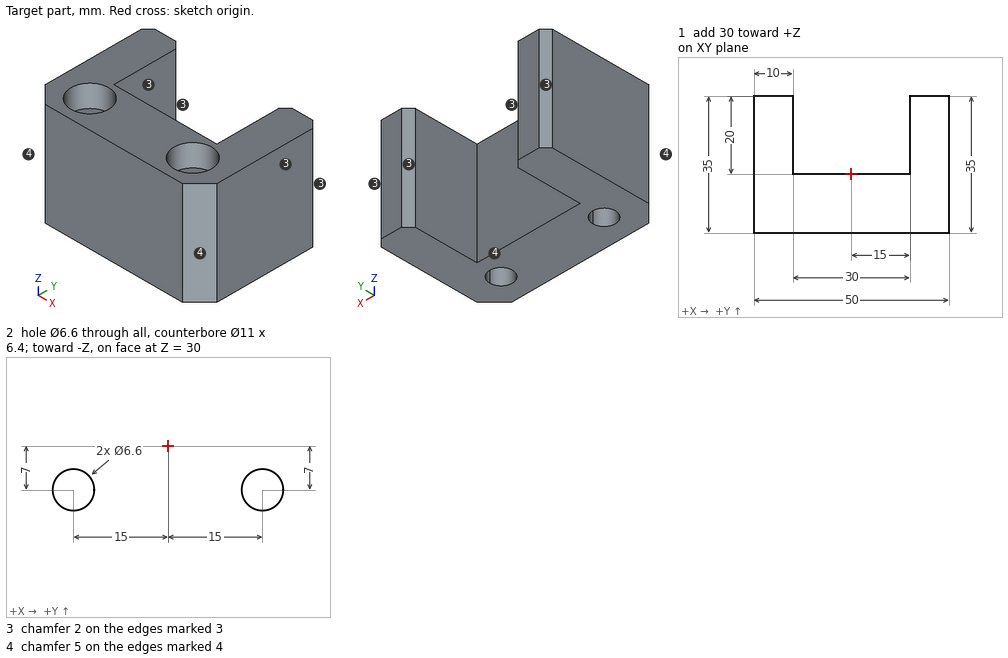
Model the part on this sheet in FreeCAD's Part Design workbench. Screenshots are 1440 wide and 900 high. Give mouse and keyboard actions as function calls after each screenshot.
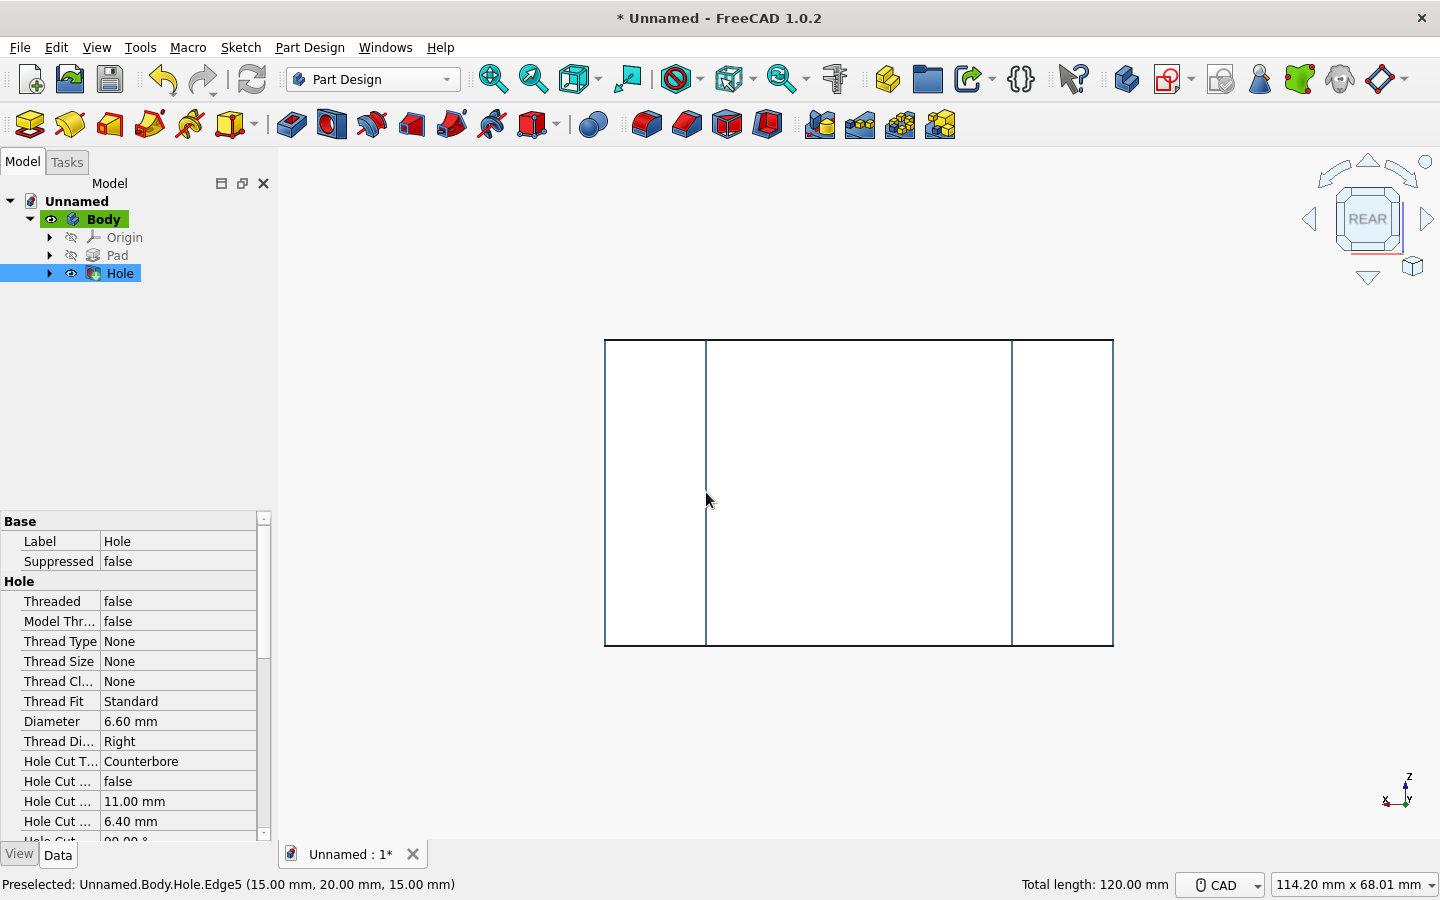
click(688, 124)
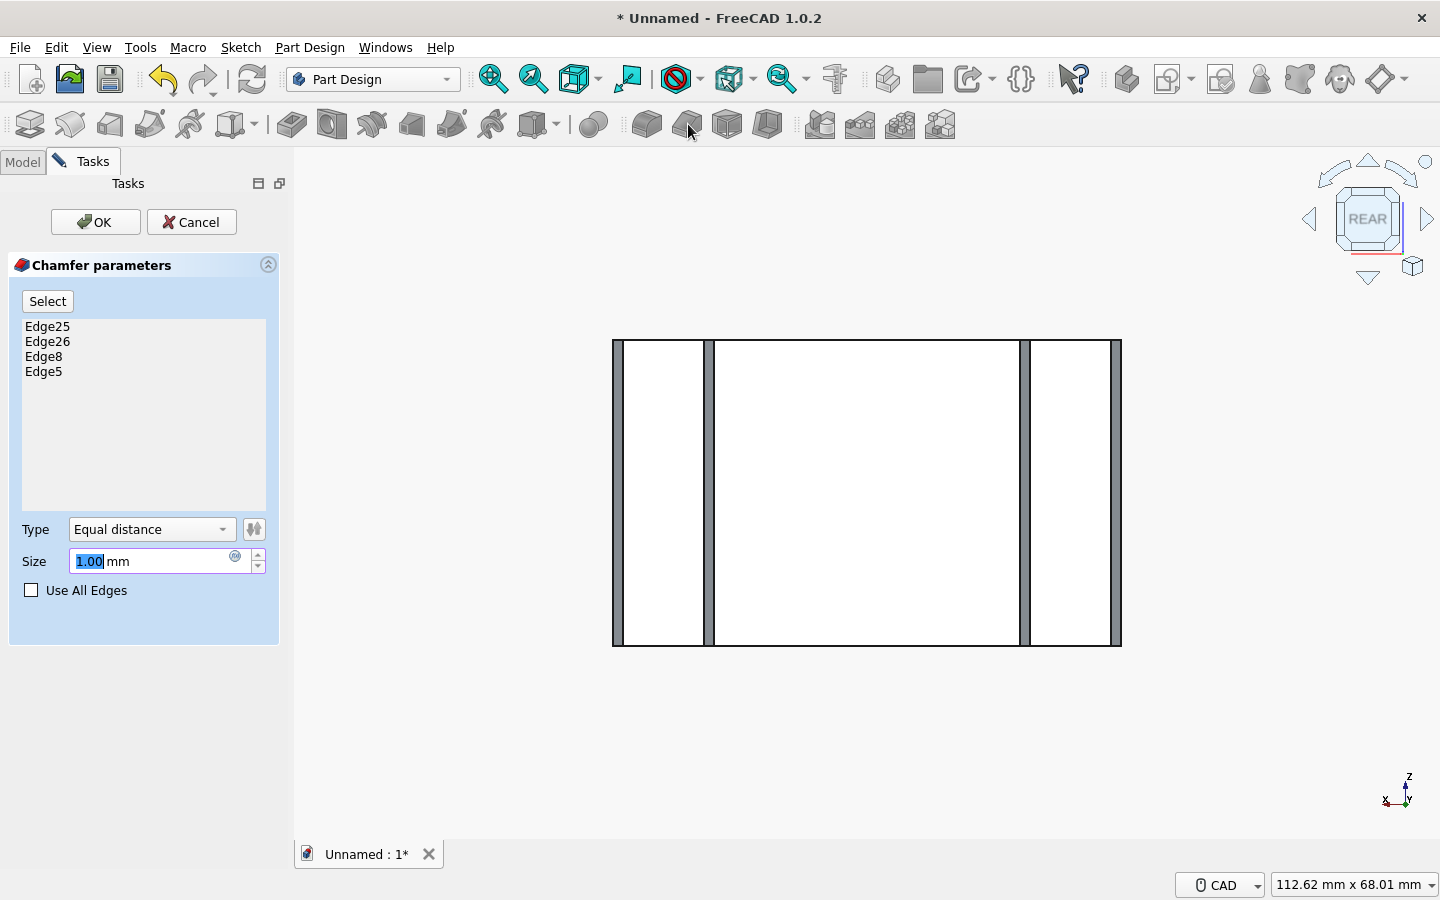
text(2)
key(Tab)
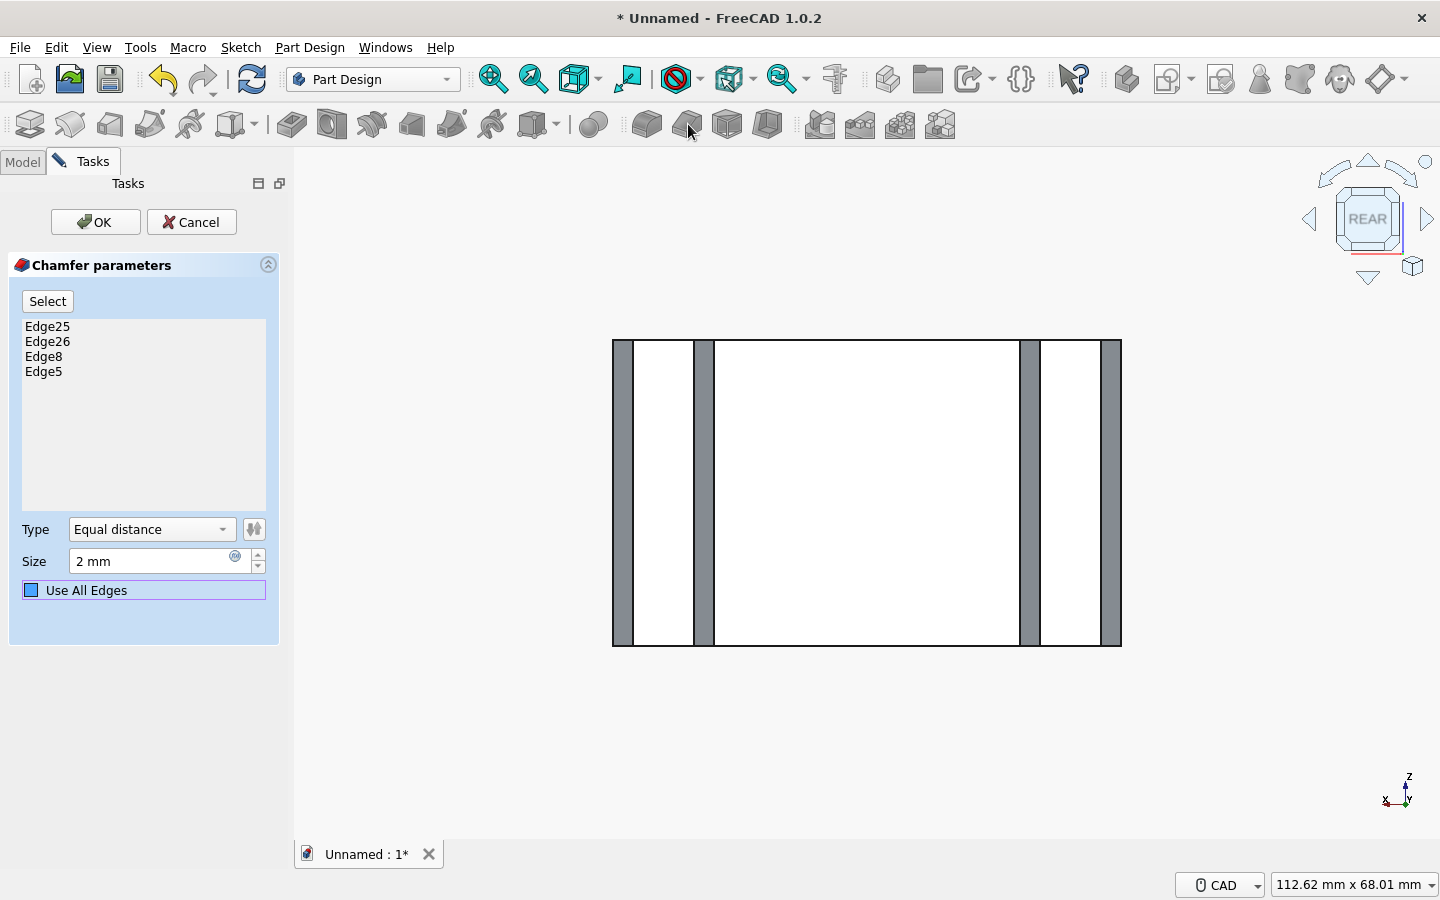
click(96, 222)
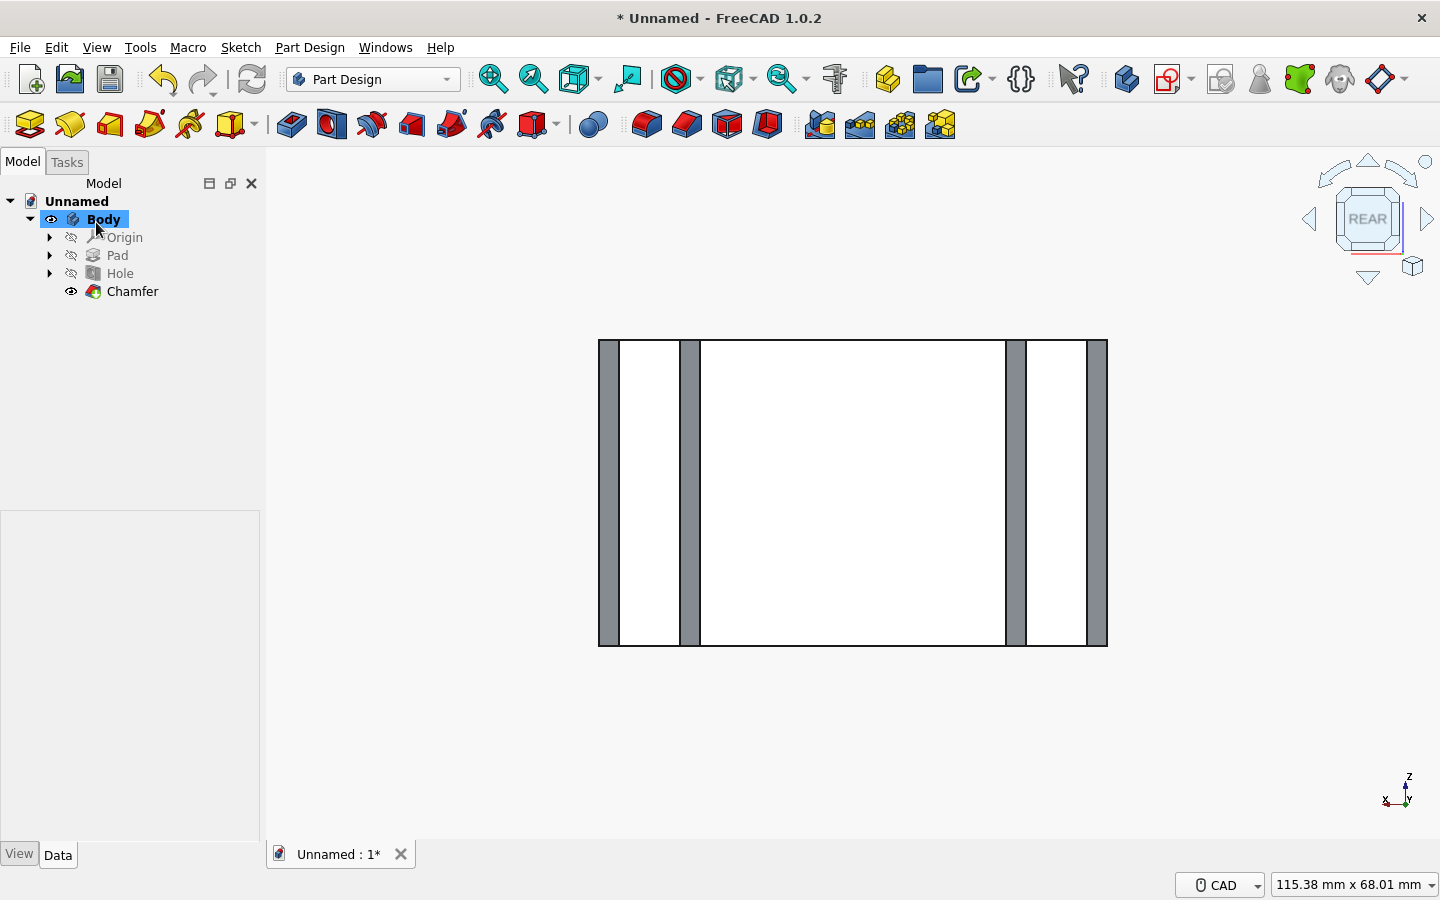
click(494, 80)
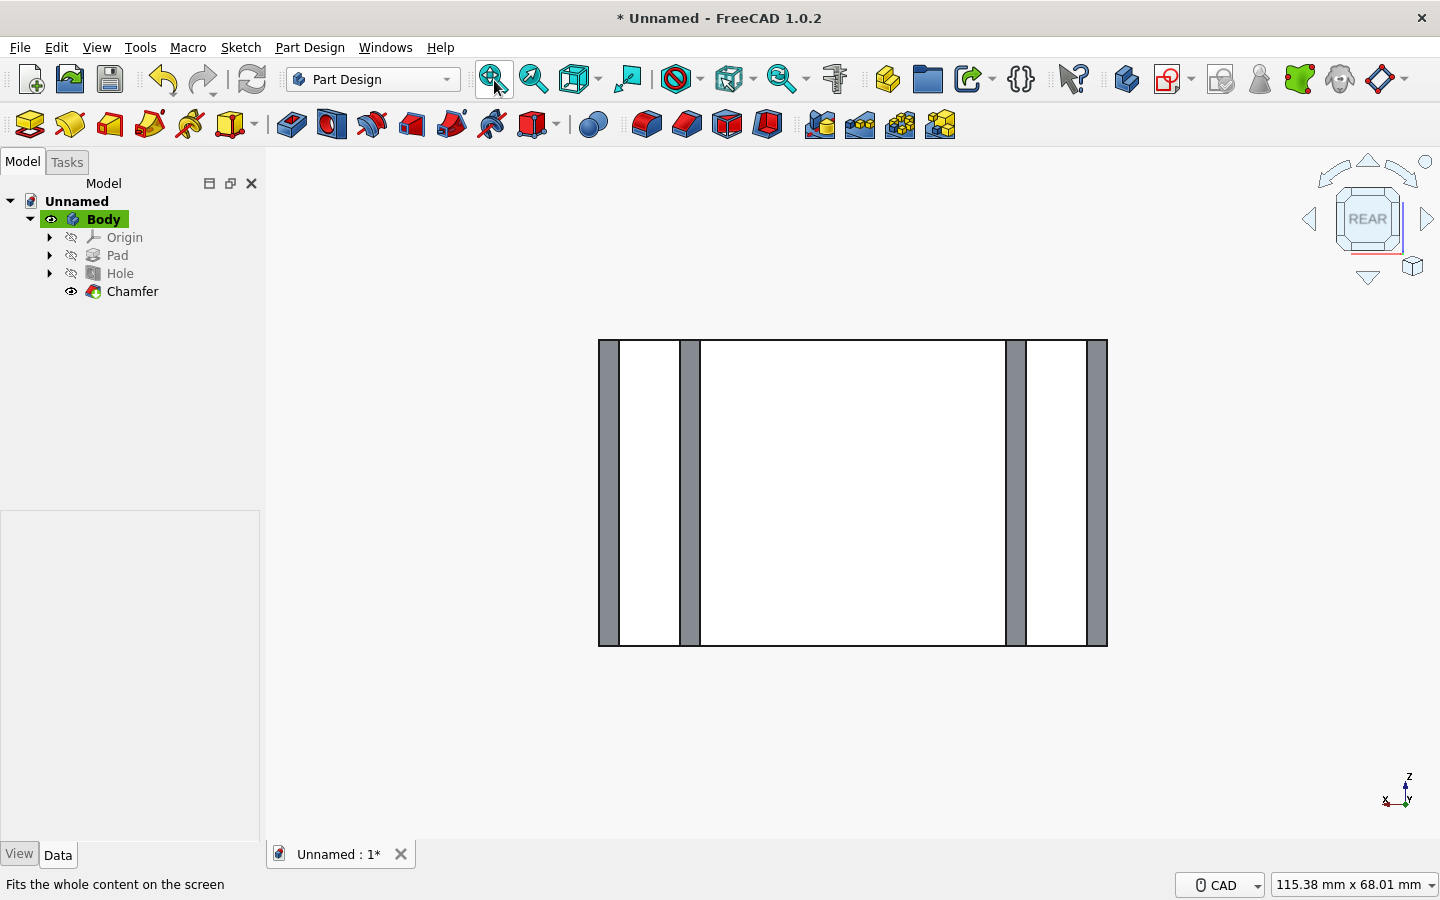
key(0)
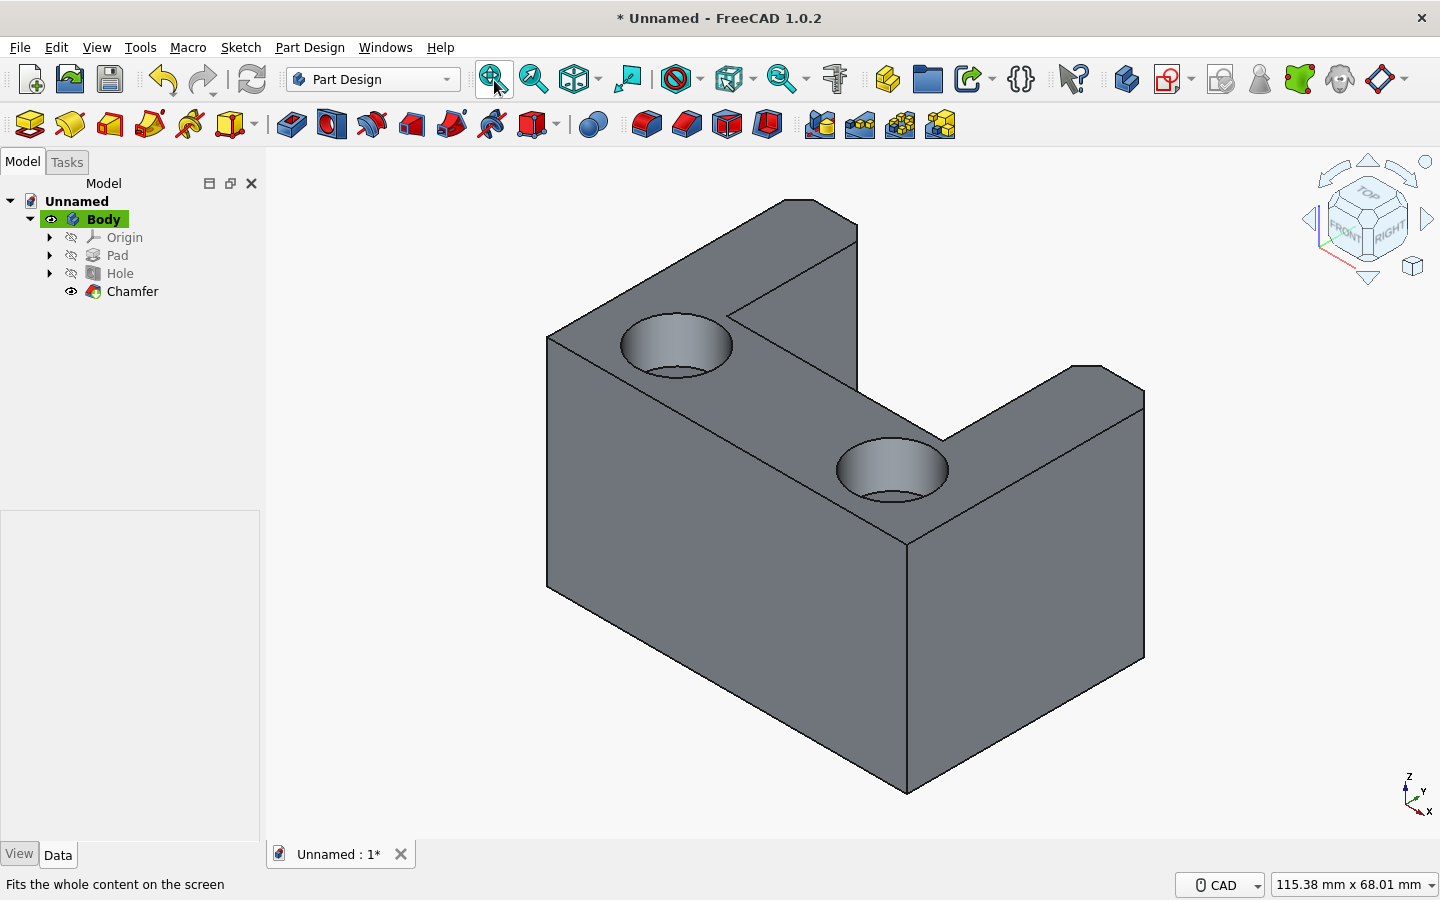
click(907, 669)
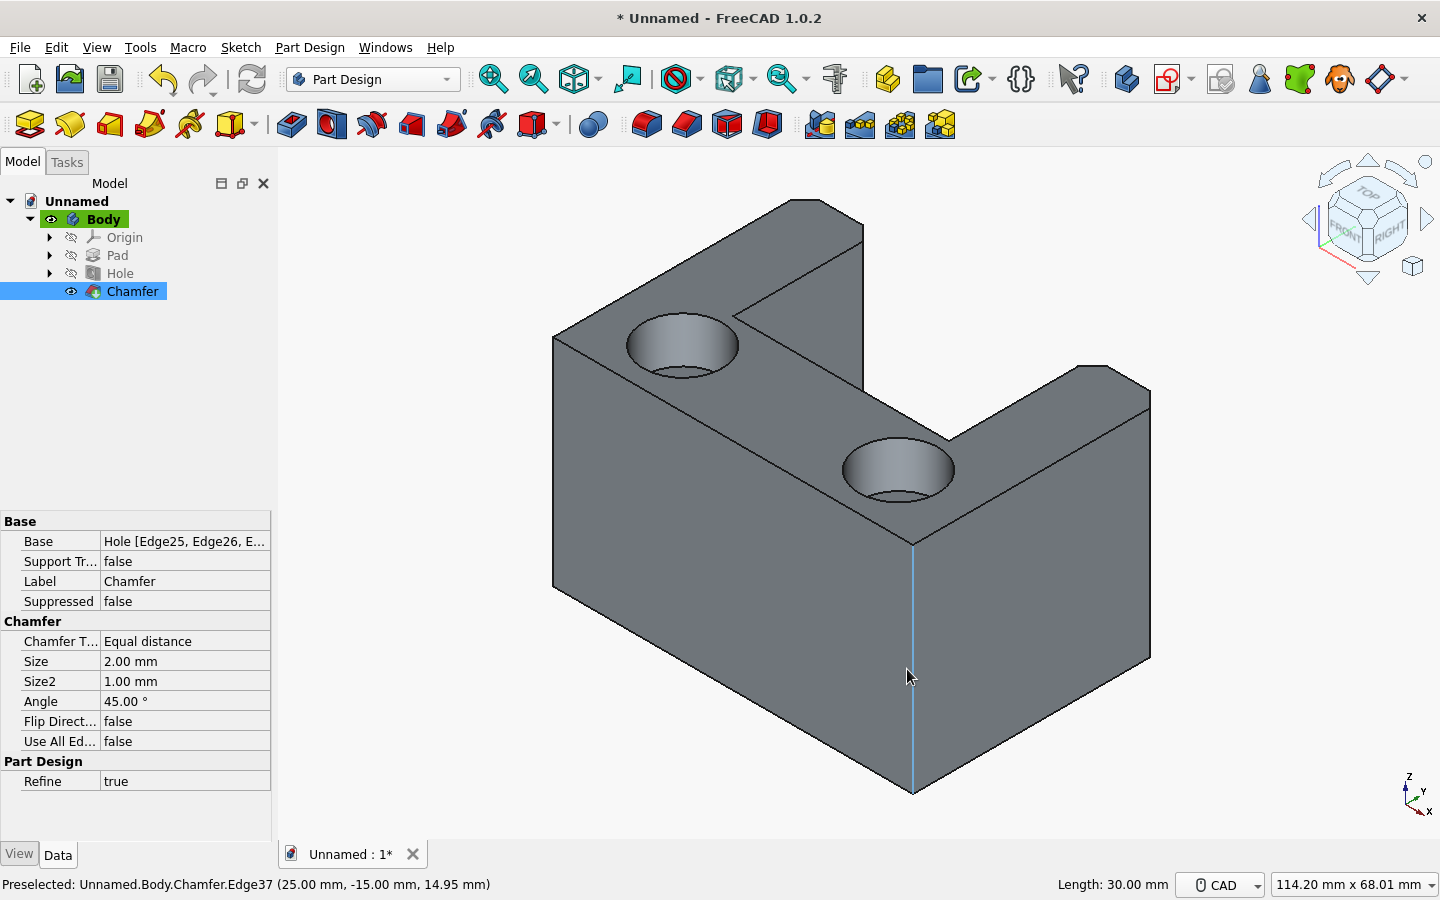
key(2)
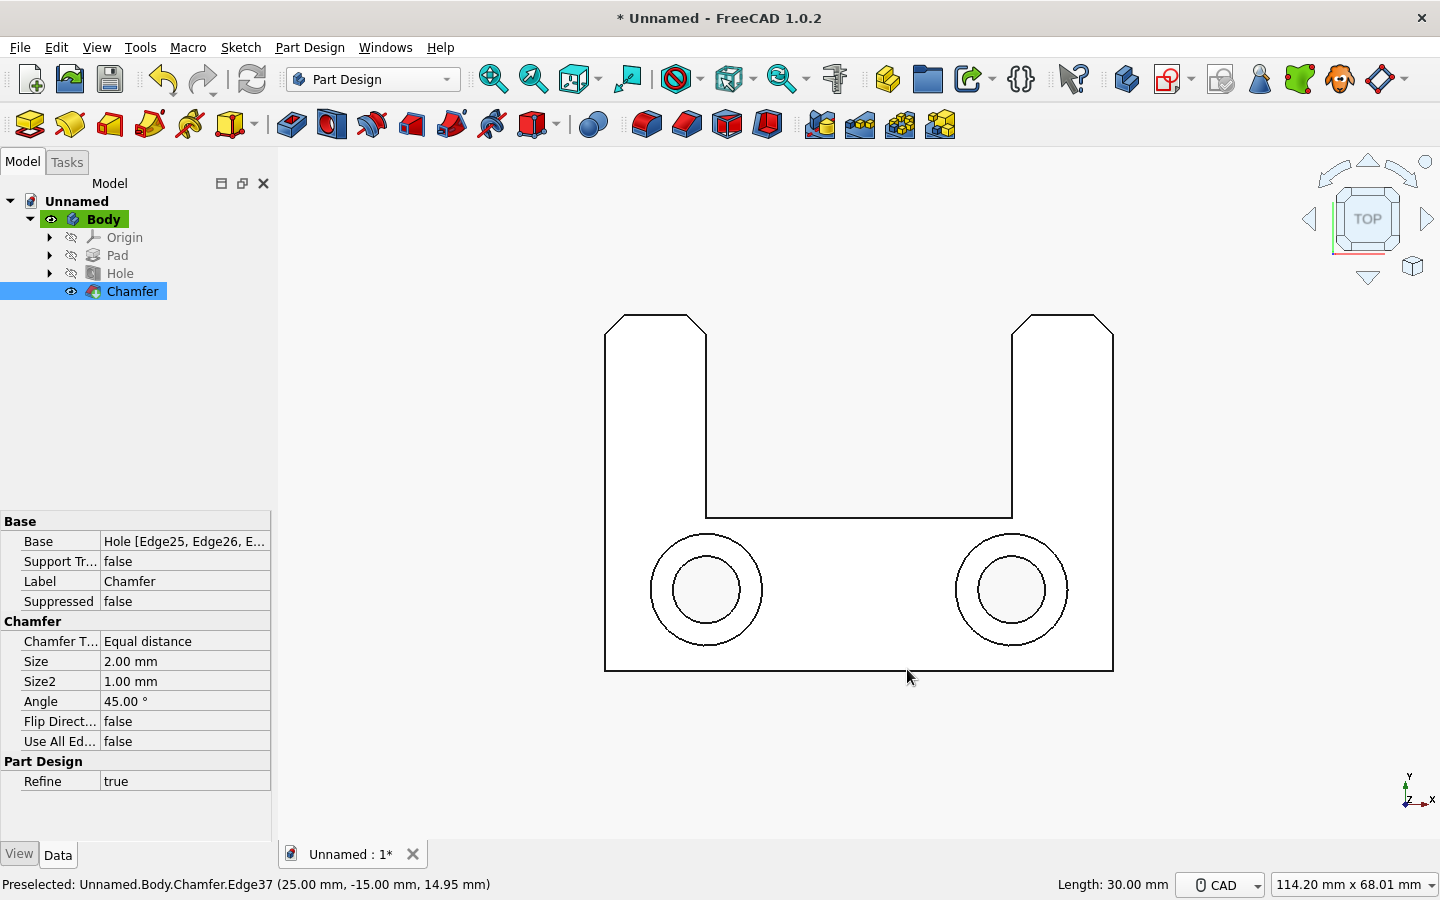
key(1)